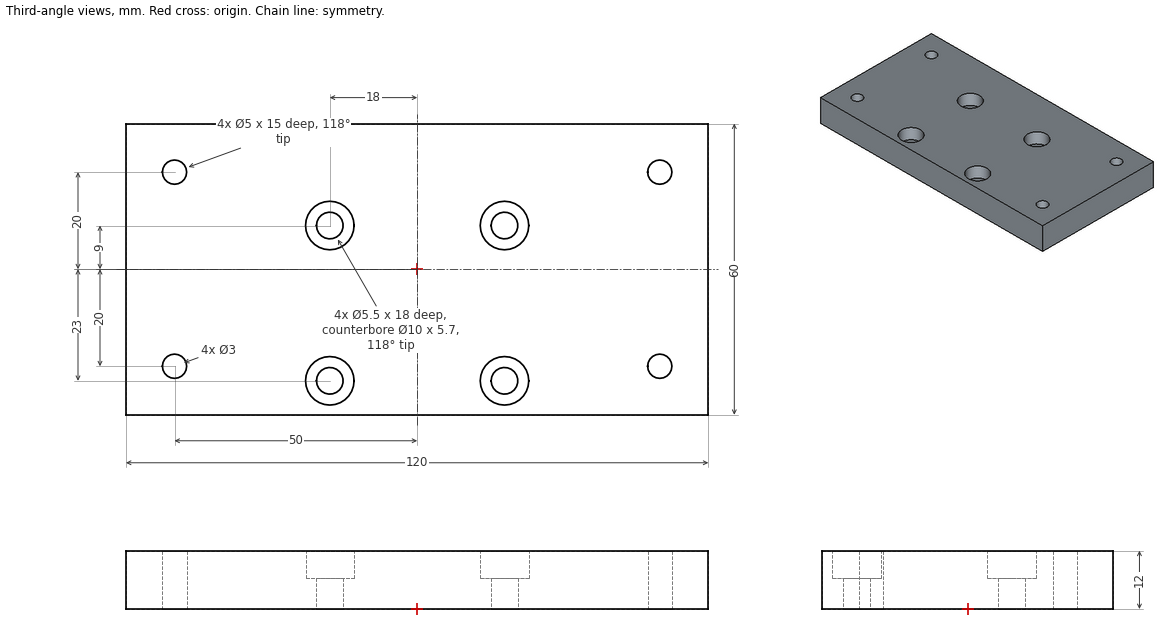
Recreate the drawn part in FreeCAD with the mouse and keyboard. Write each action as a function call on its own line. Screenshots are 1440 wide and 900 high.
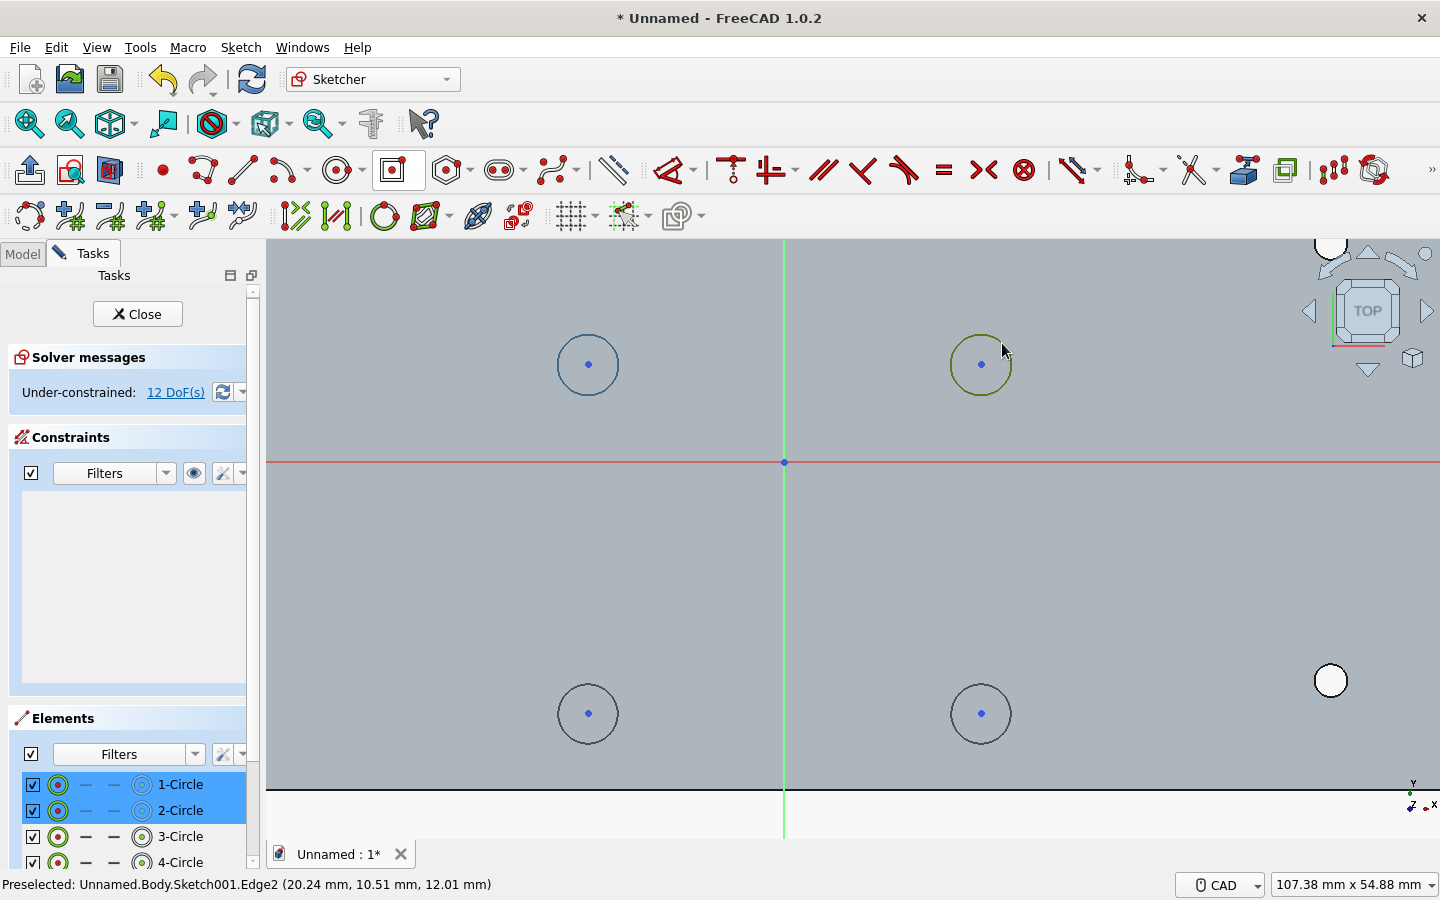
click(609, 693)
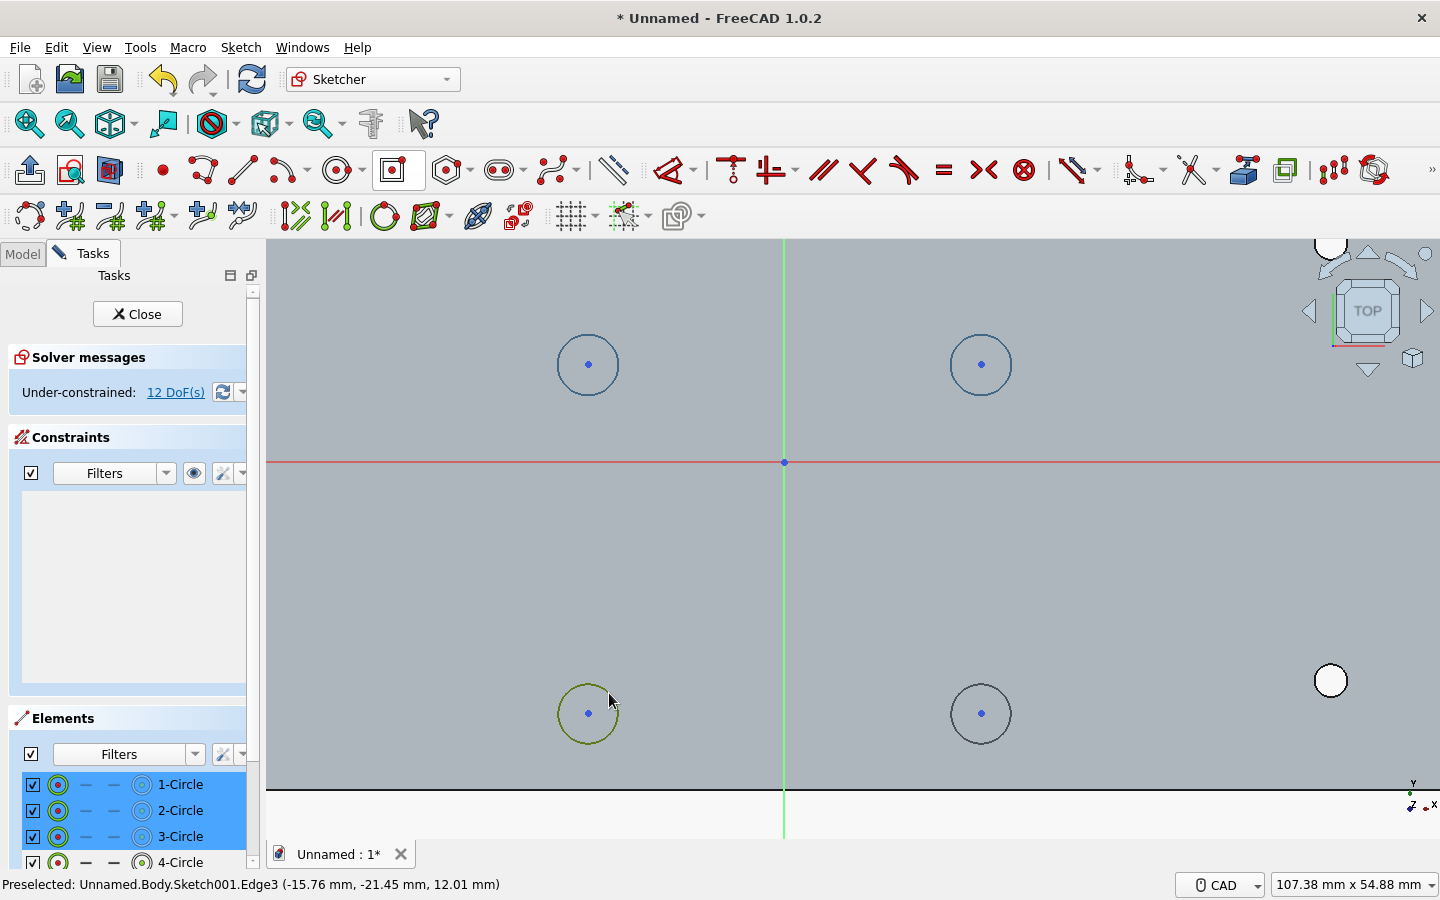
click(1002, 693)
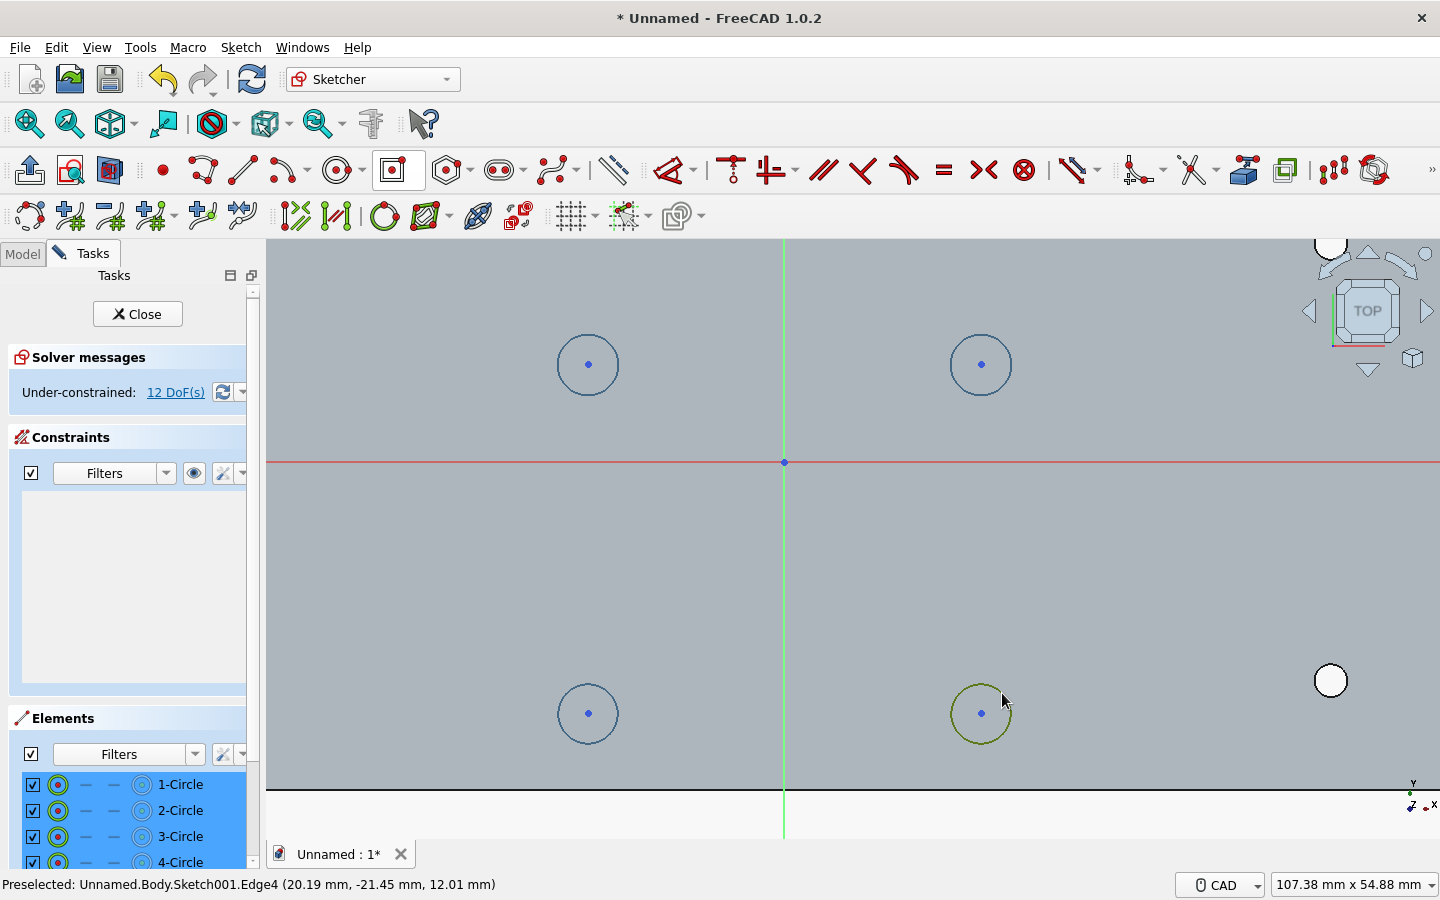
click(944, 170)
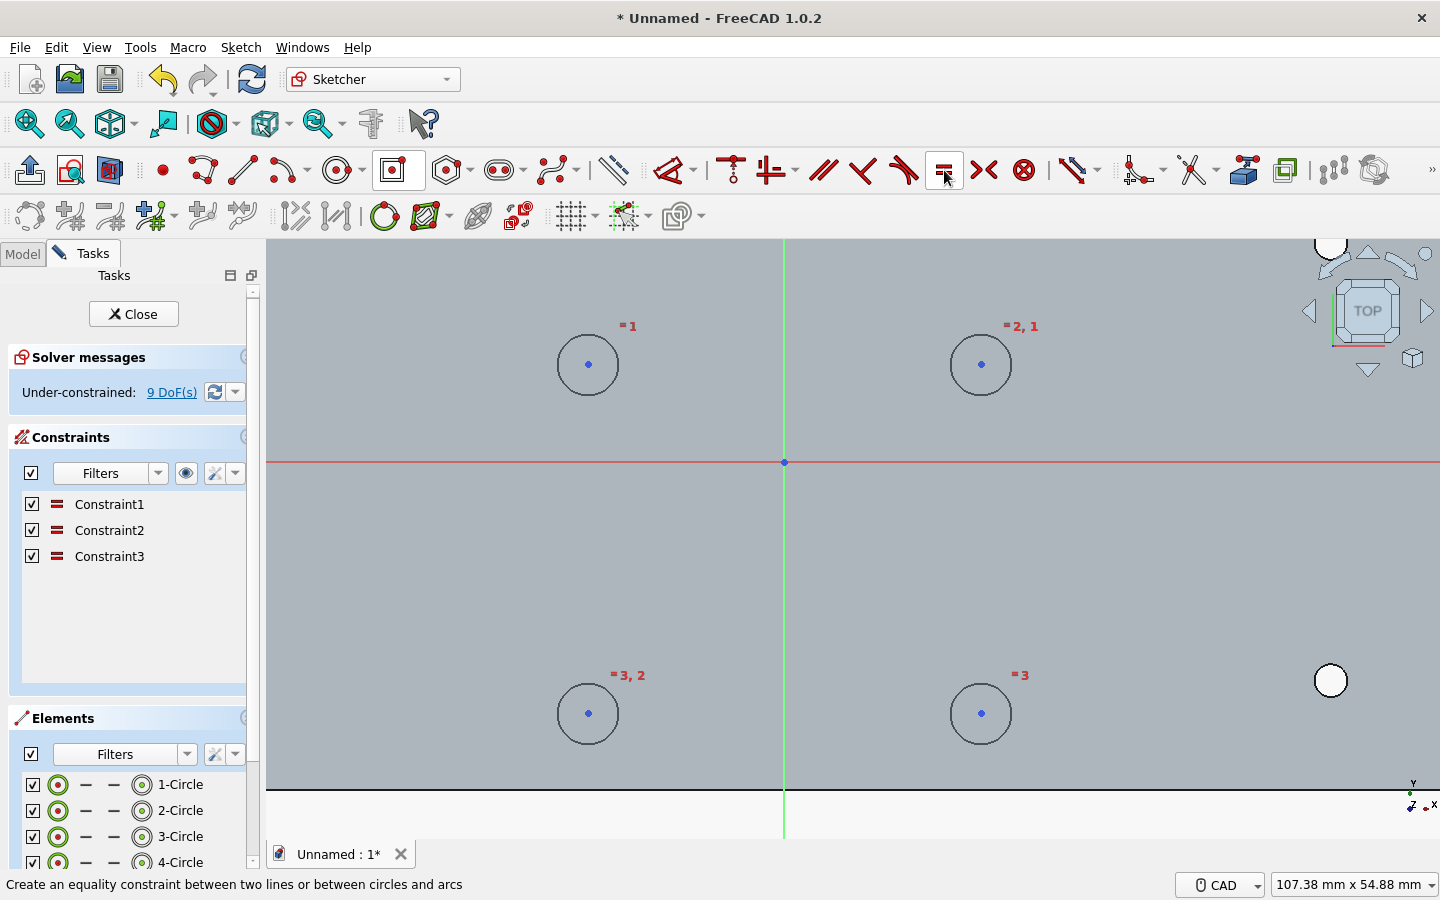
click(588, 365)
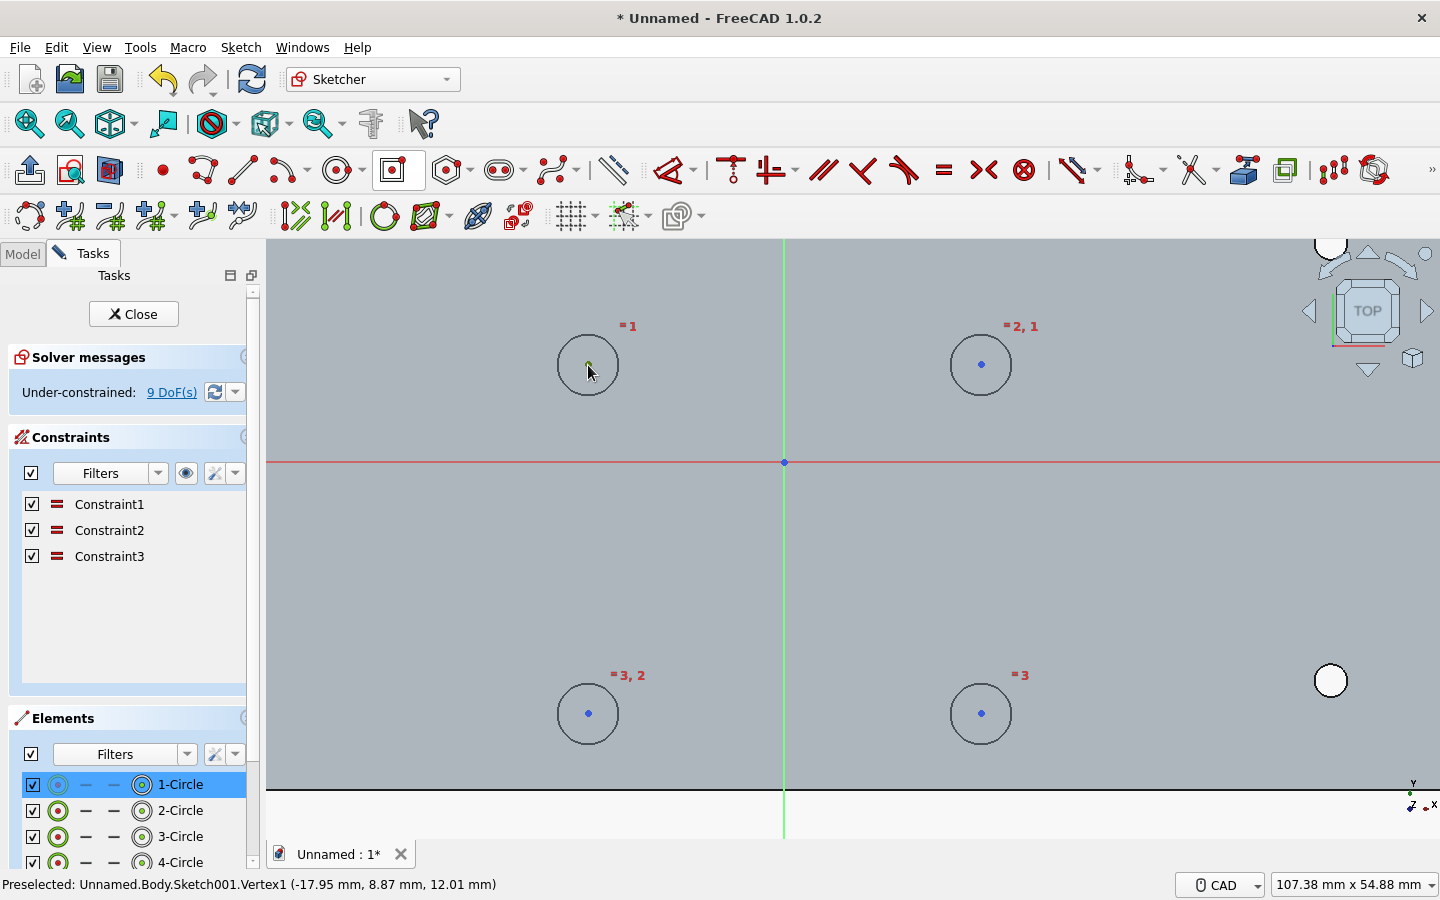
click(981, 365)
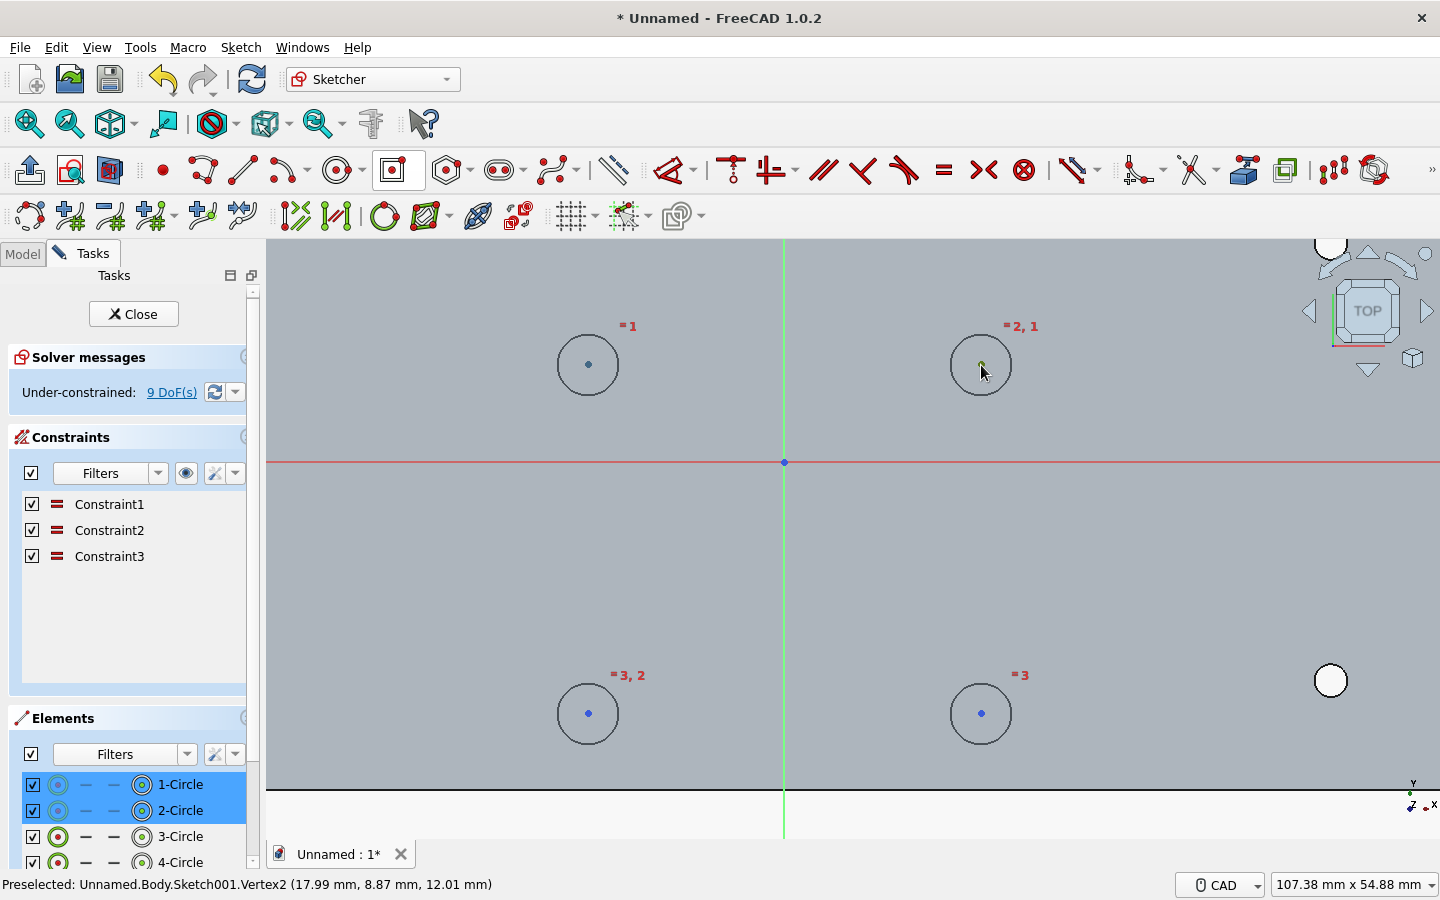
click(784, 772)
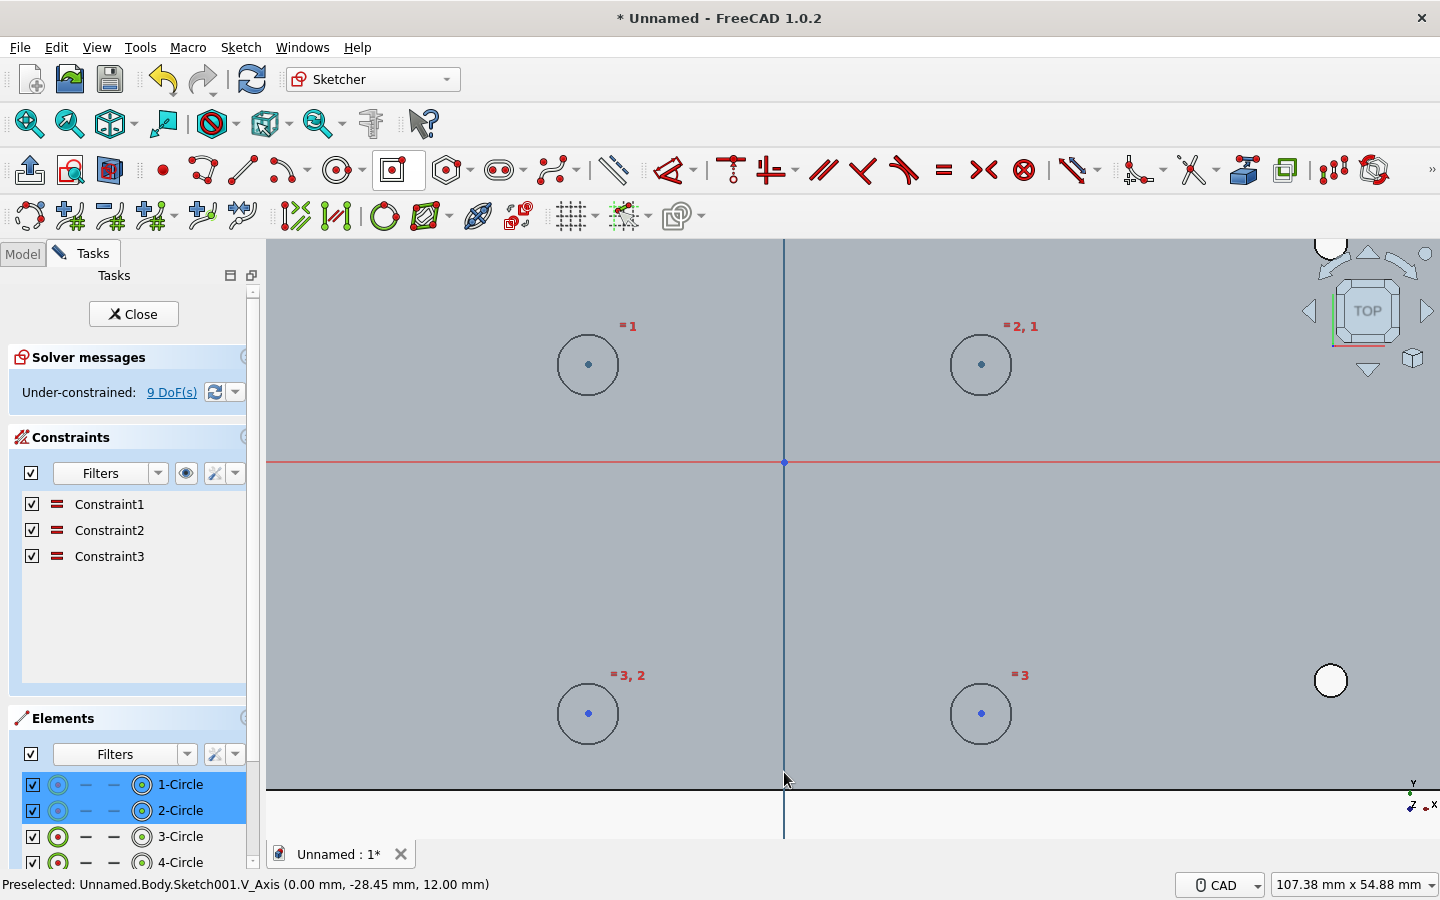
click(984, 170)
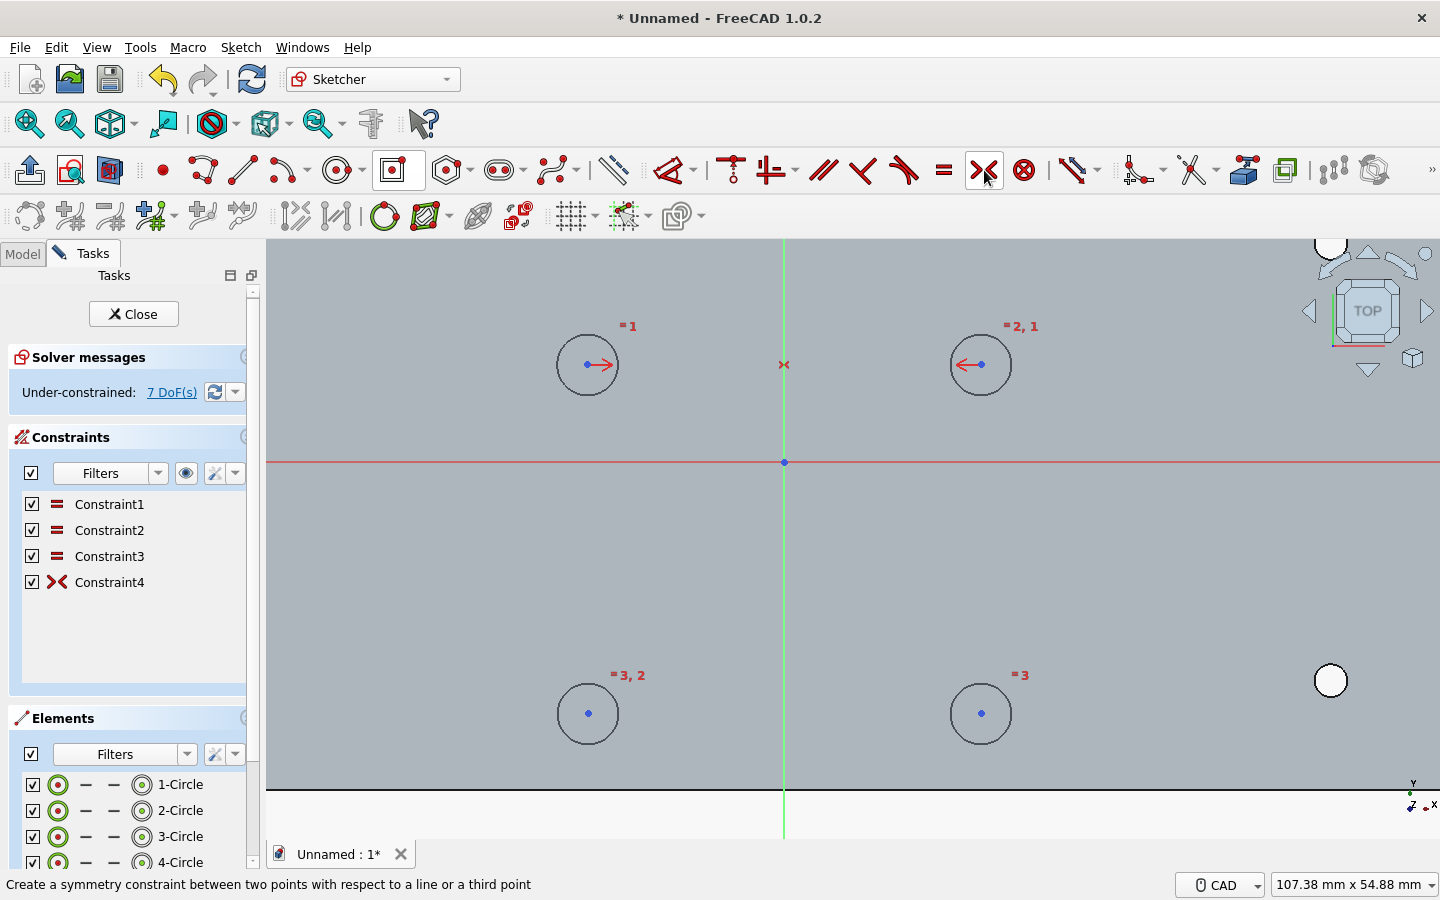
click(588, 714)